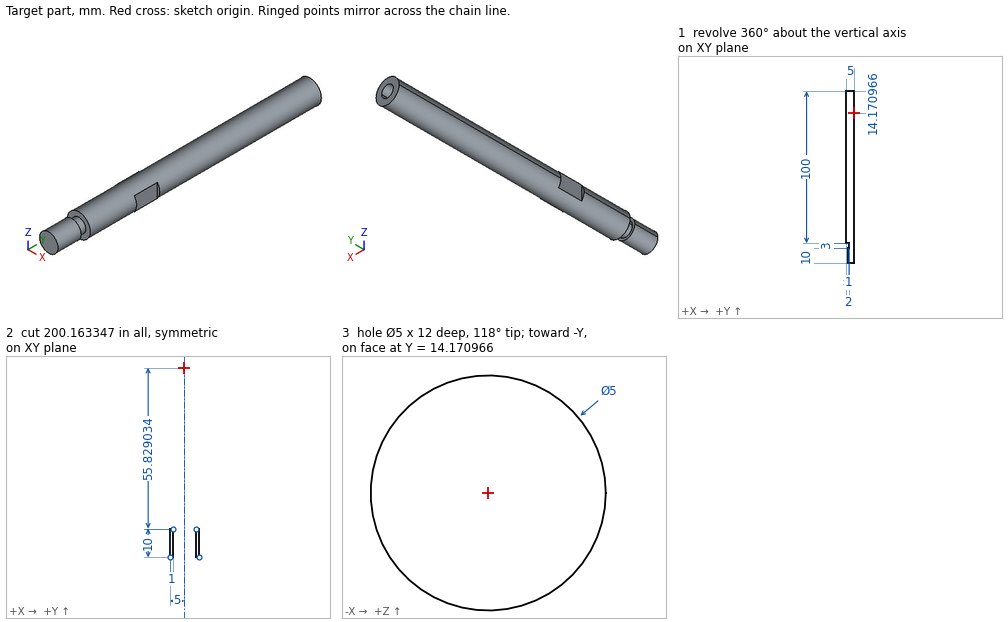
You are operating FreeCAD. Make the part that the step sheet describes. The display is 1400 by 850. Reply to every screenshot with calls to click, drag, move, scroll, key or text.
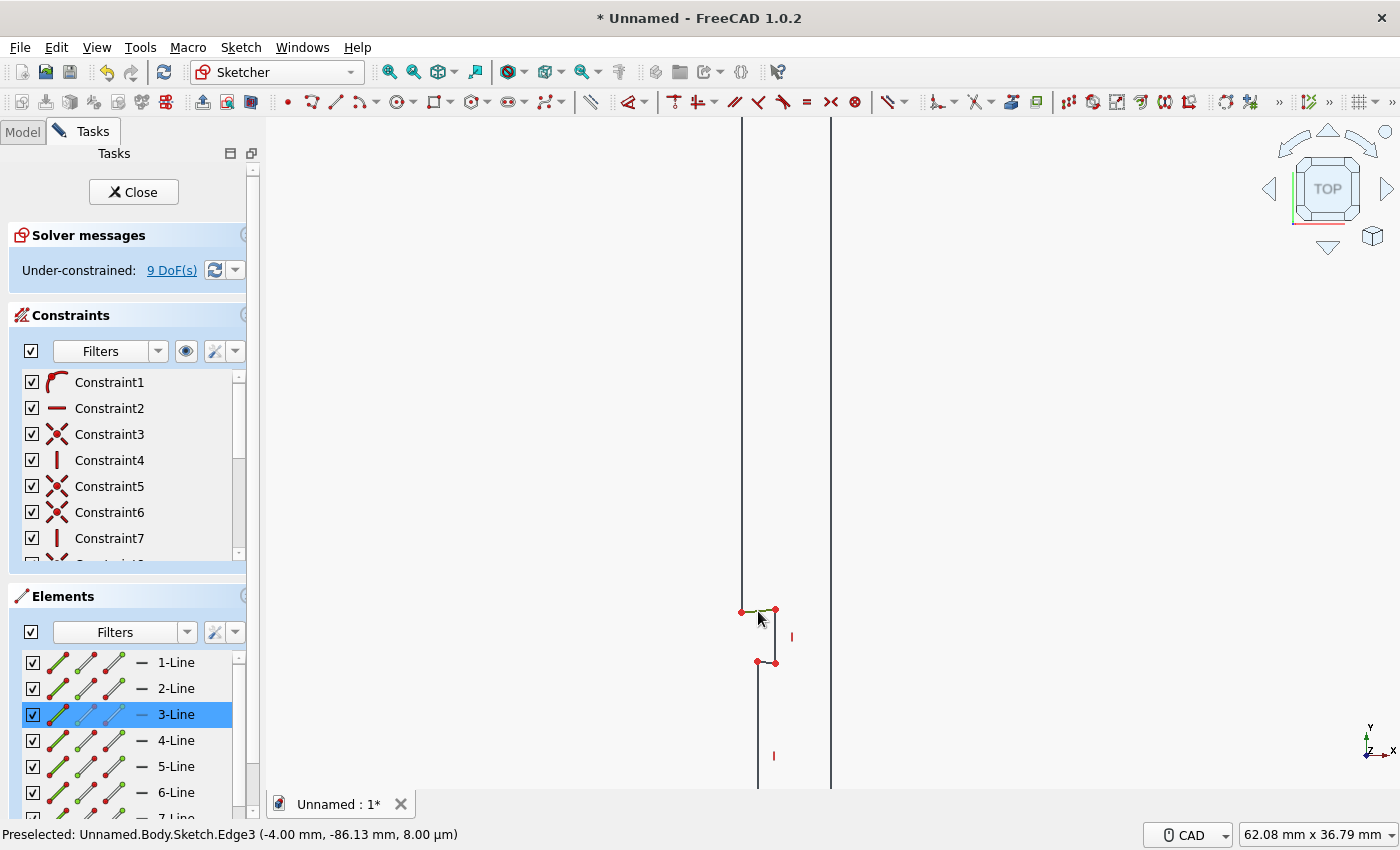
click(716, 102)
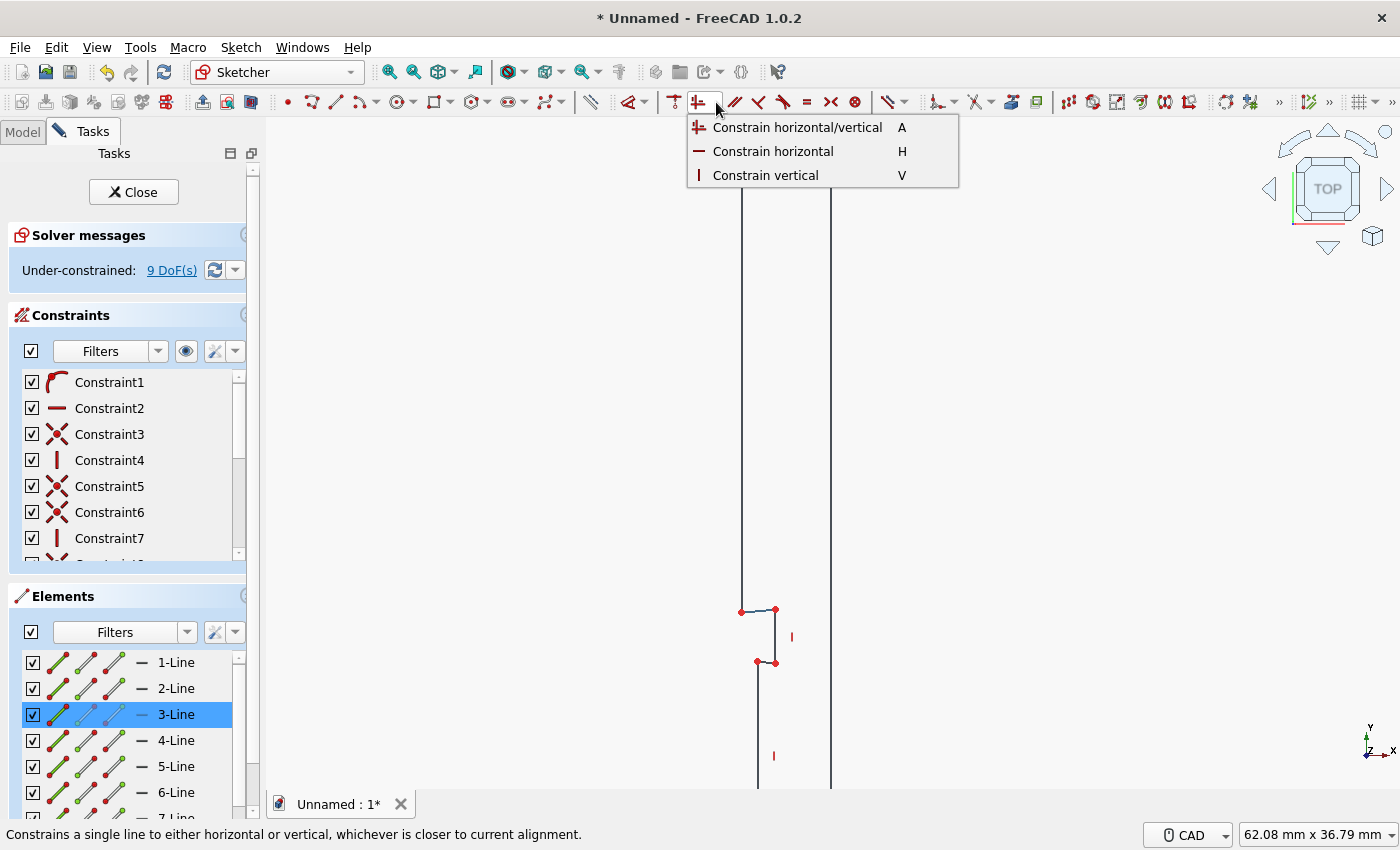
click(823, 151)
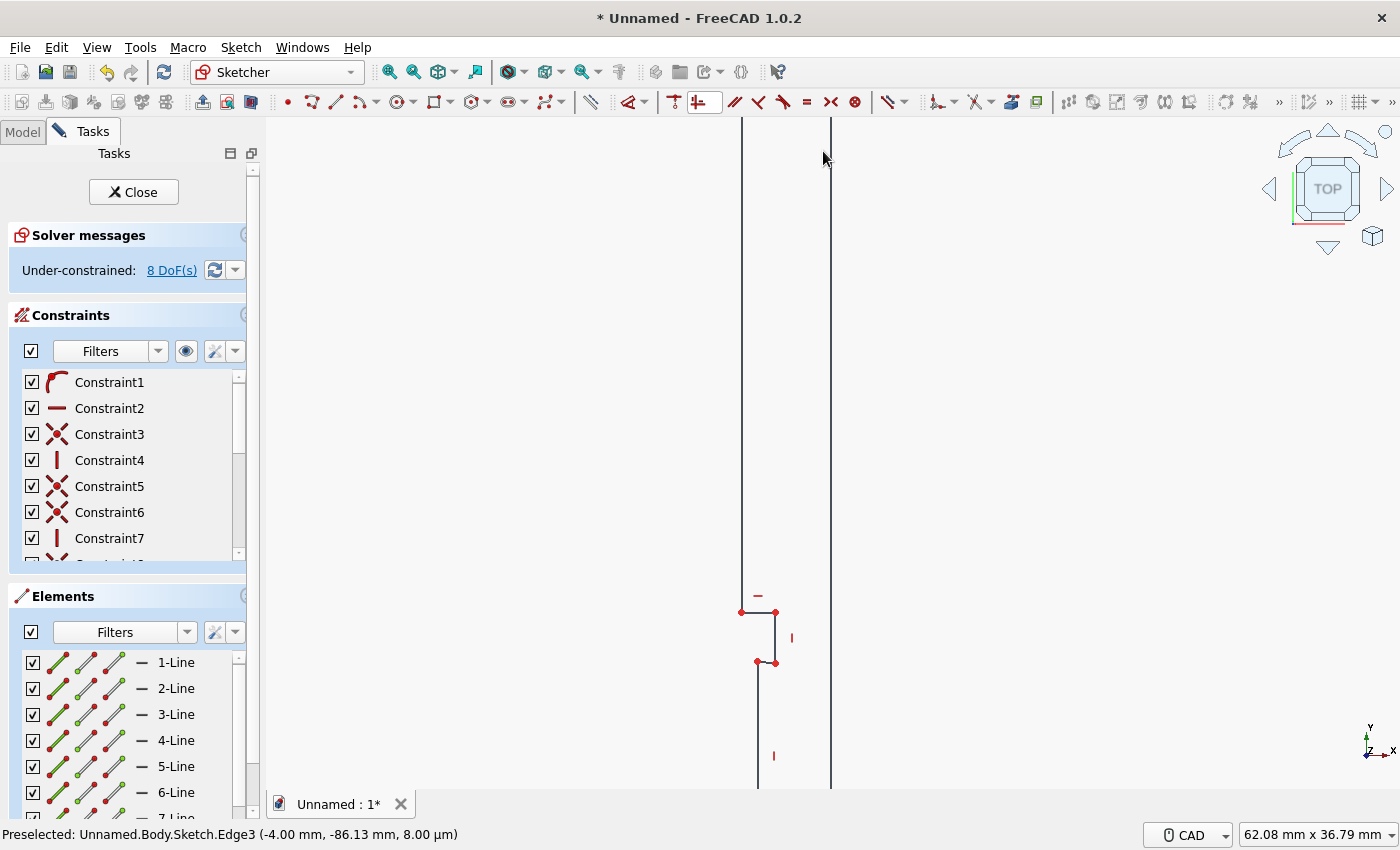
scroll(767, 663, up, 3)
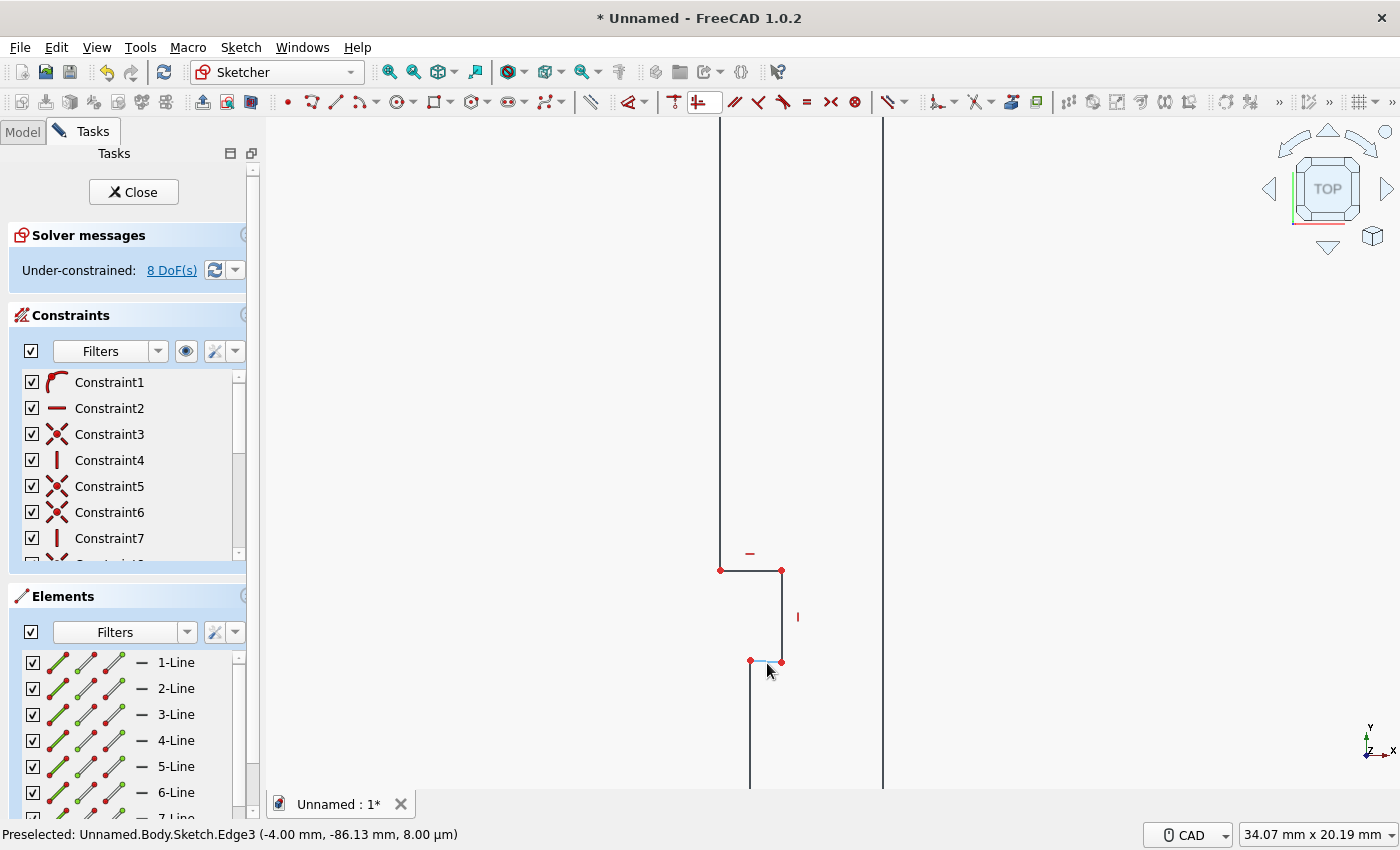
click(766, 661)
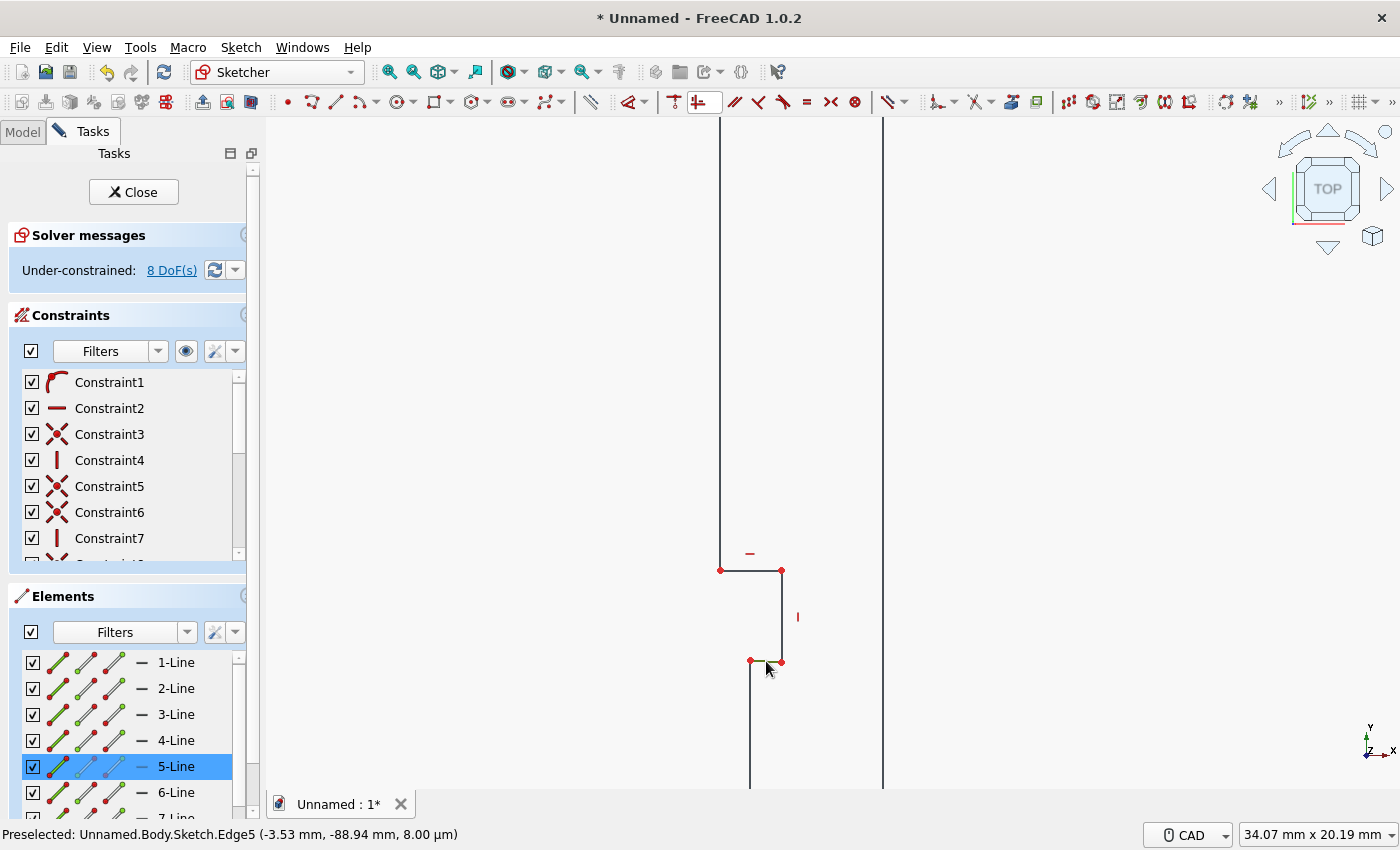
key(h)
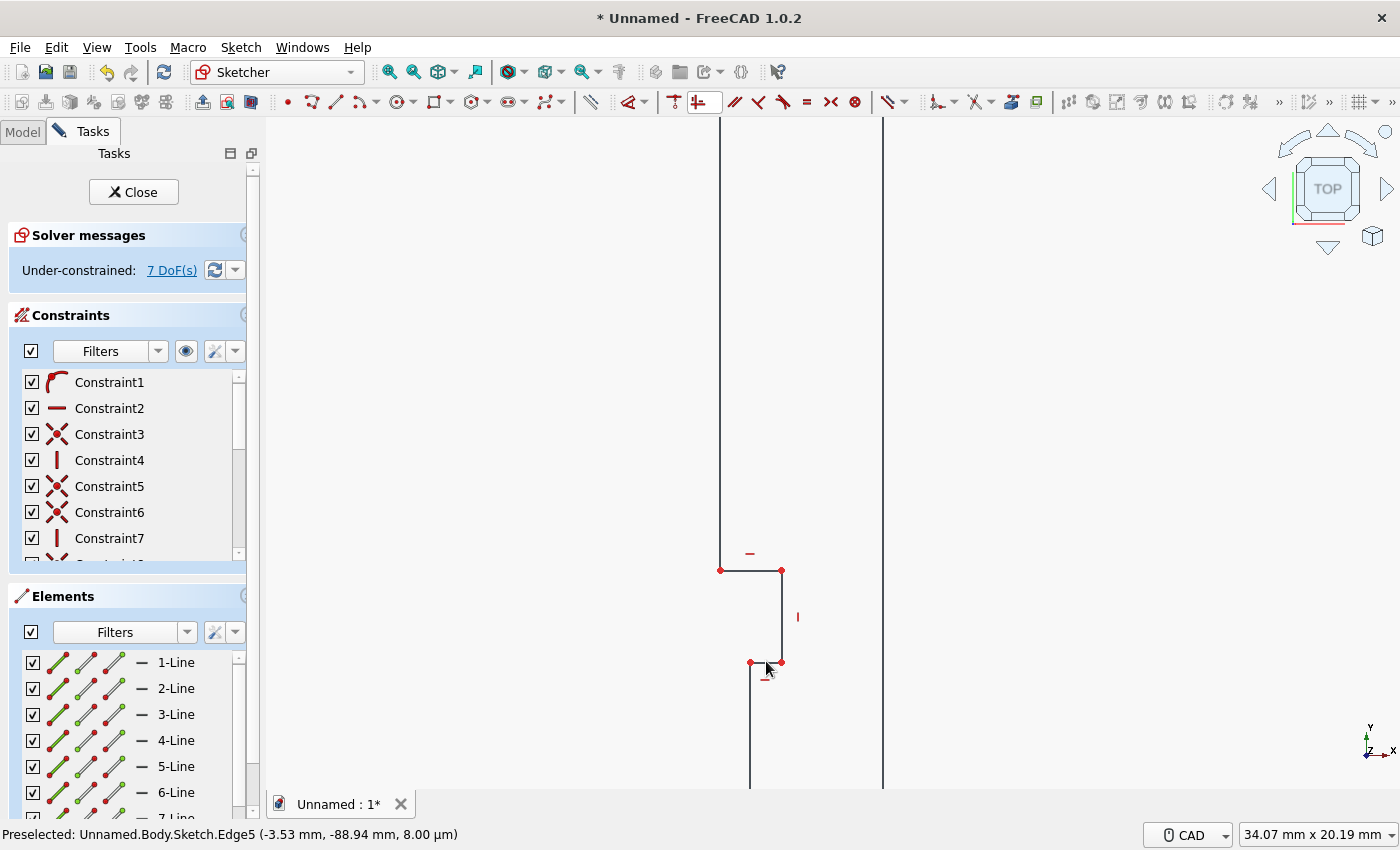
click(628, 102)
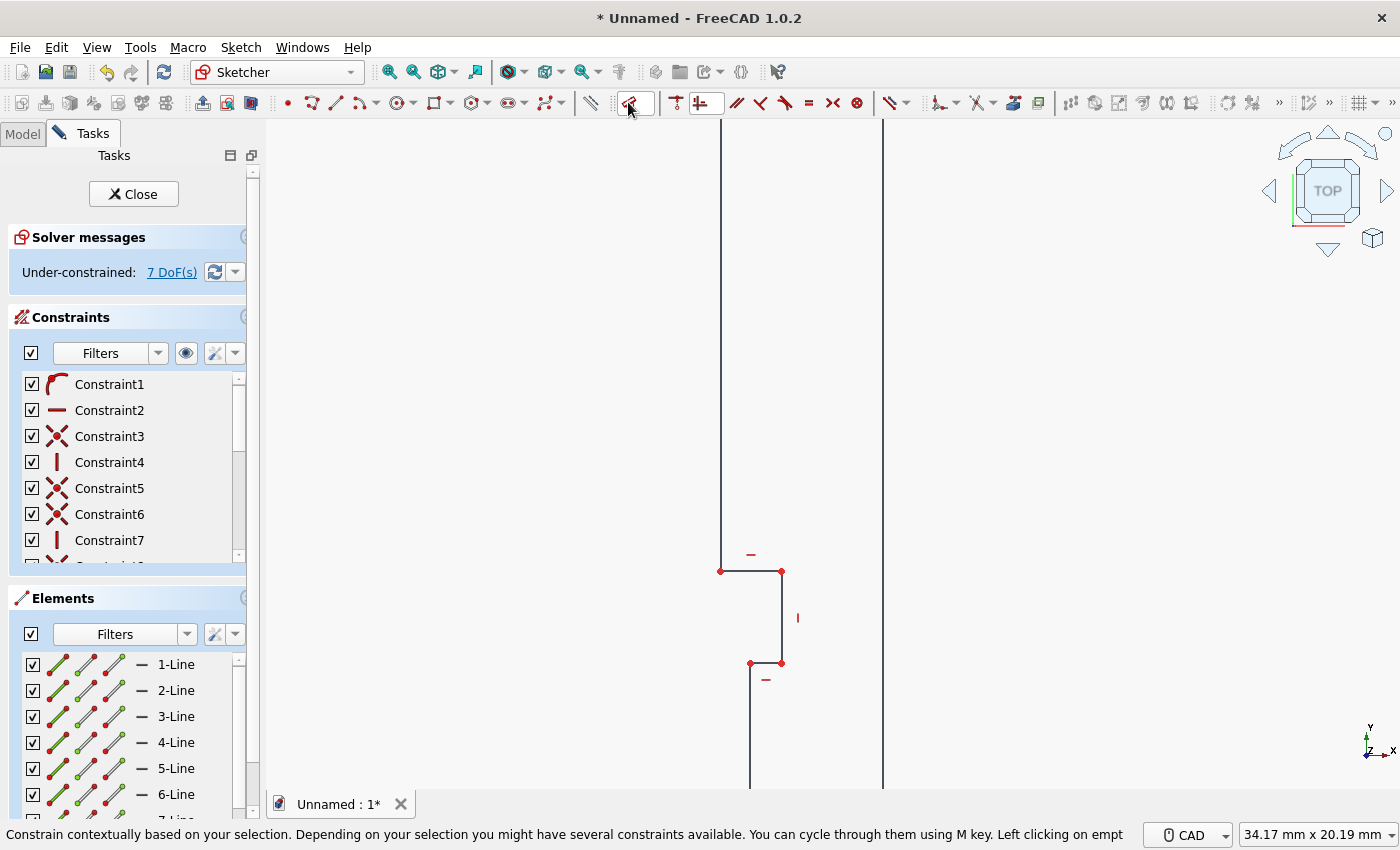
scroll(760, 621, down, 11)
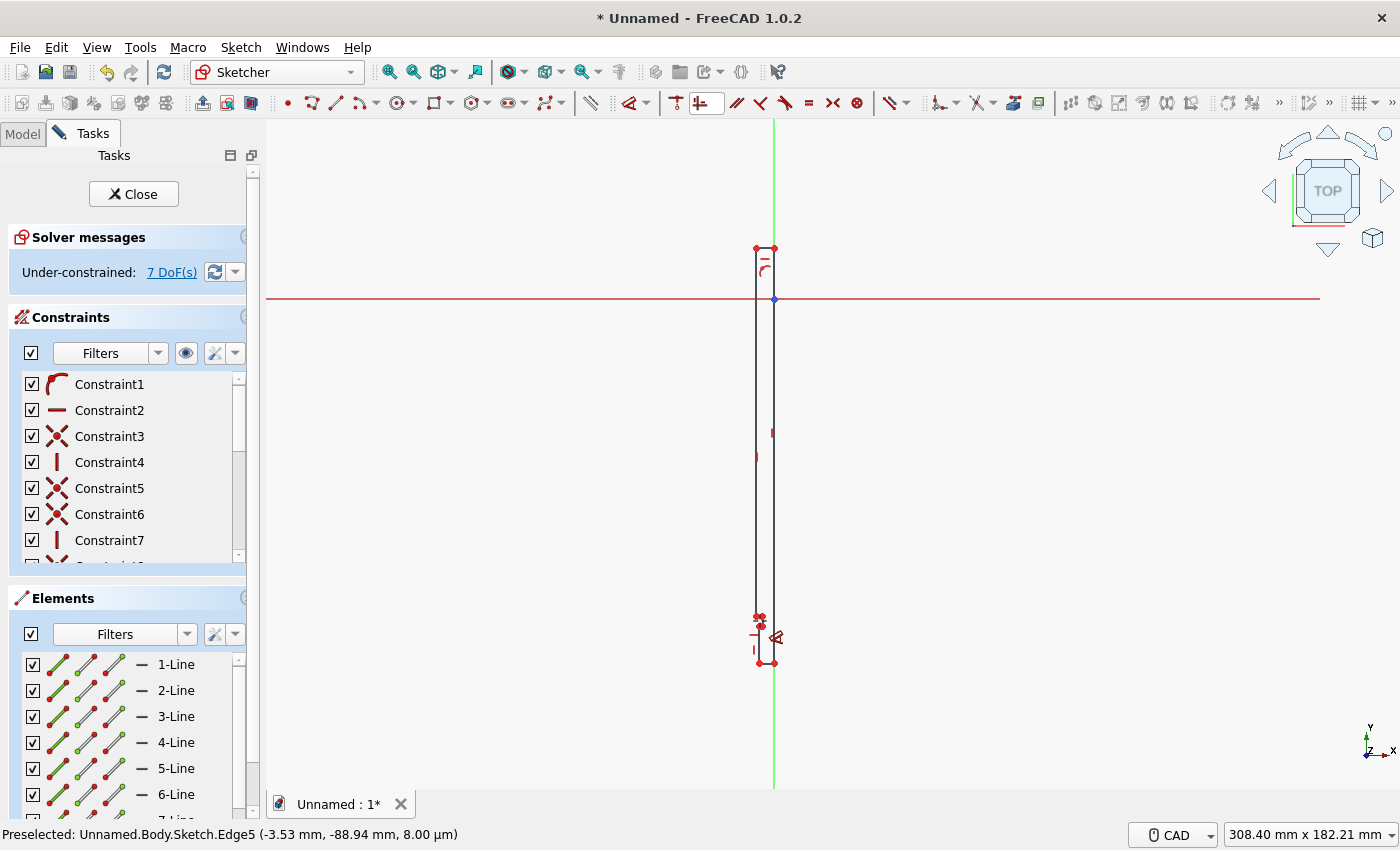
scroll(769, 248, up, 5)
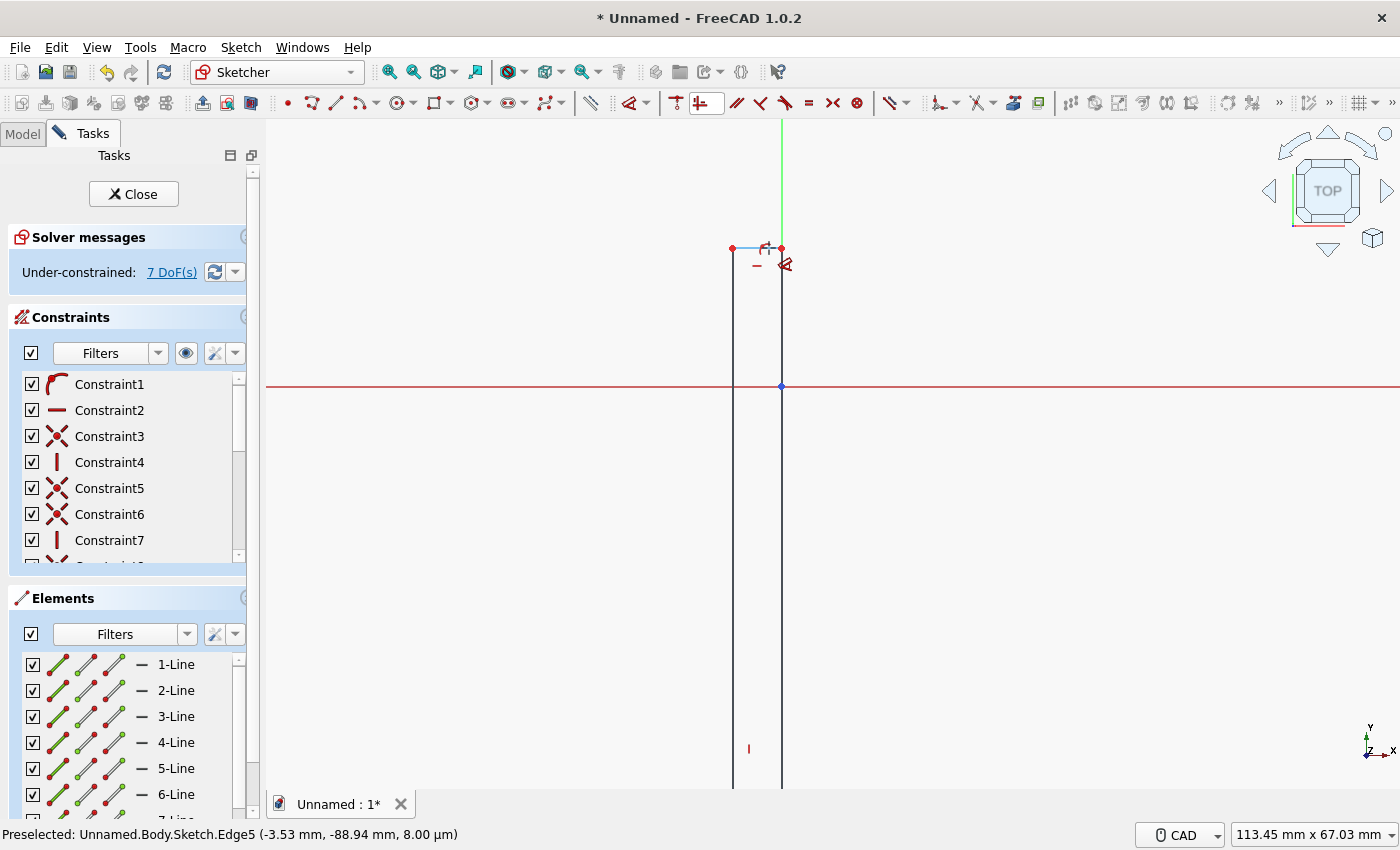
click(767, 248)
click(757, 214)